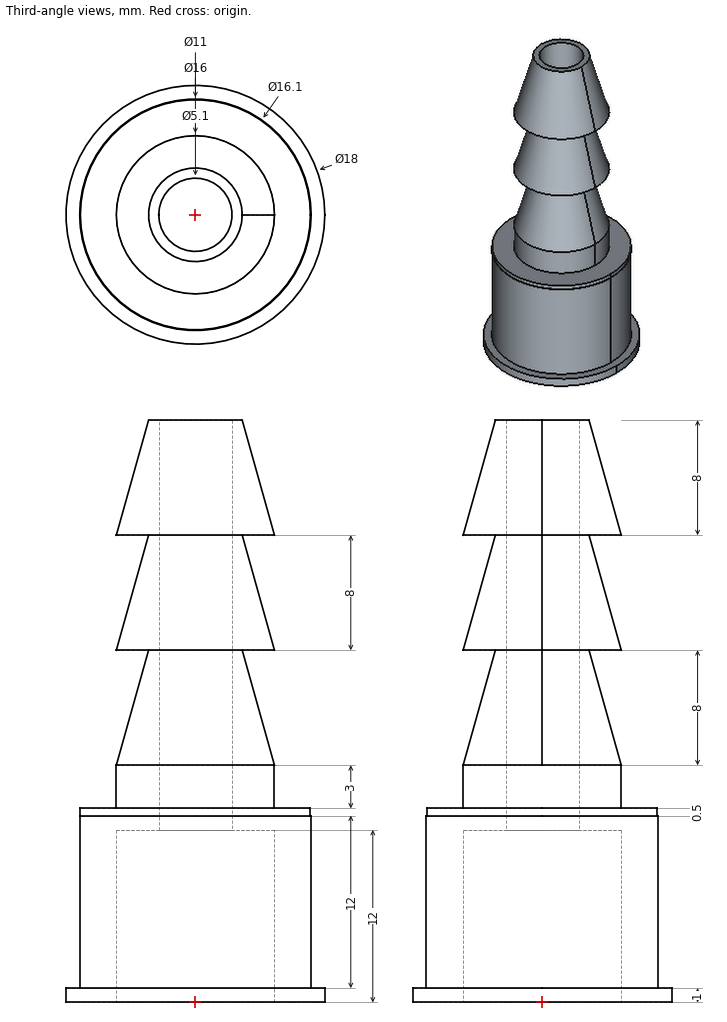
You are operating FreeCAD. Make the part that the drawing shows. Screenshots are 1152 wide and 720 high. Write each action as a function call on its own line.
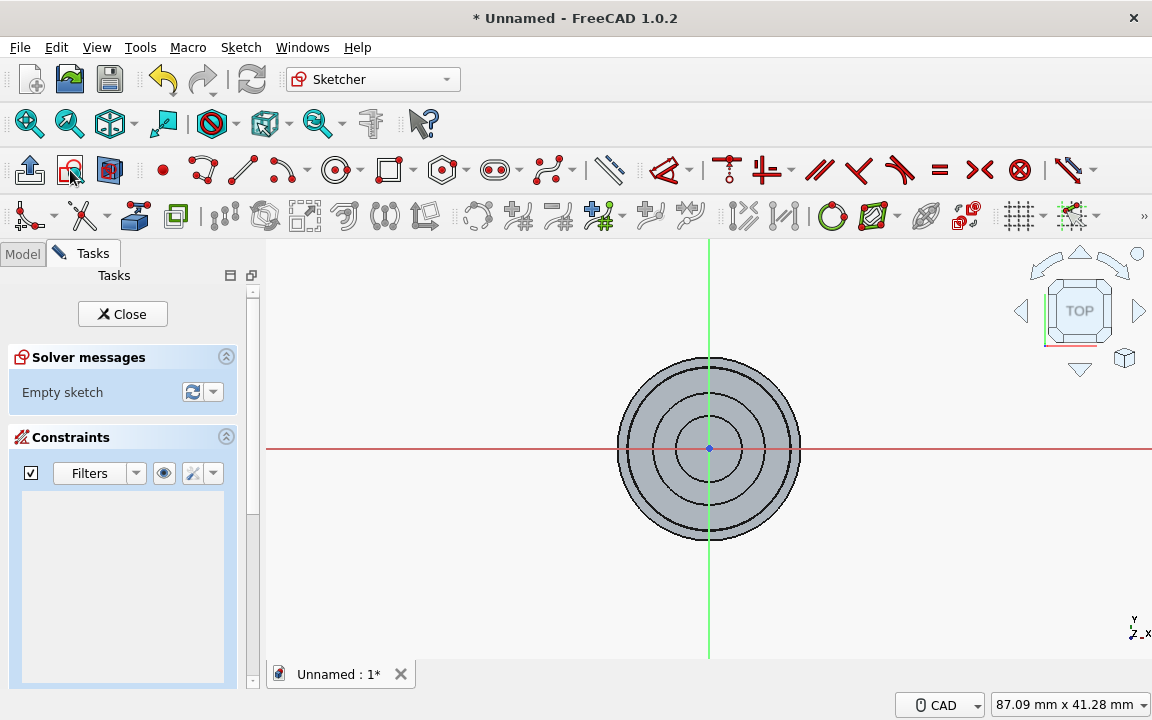
scroll(765, 449, up, 4)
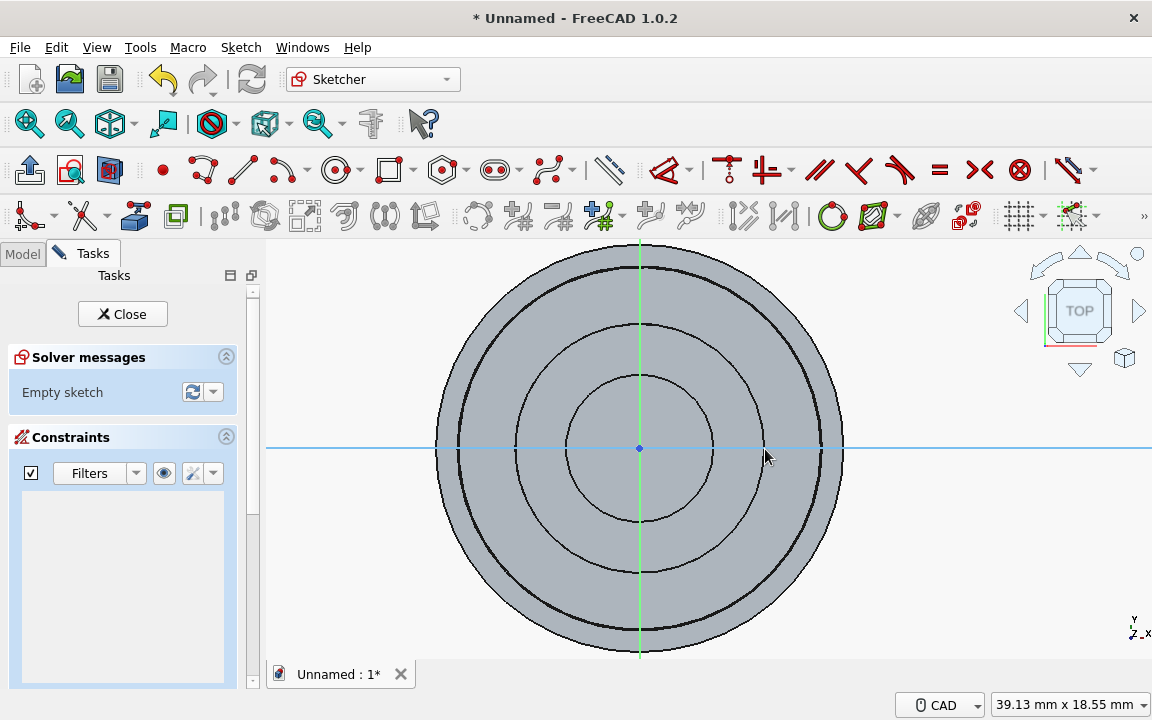
key(g)
key(c)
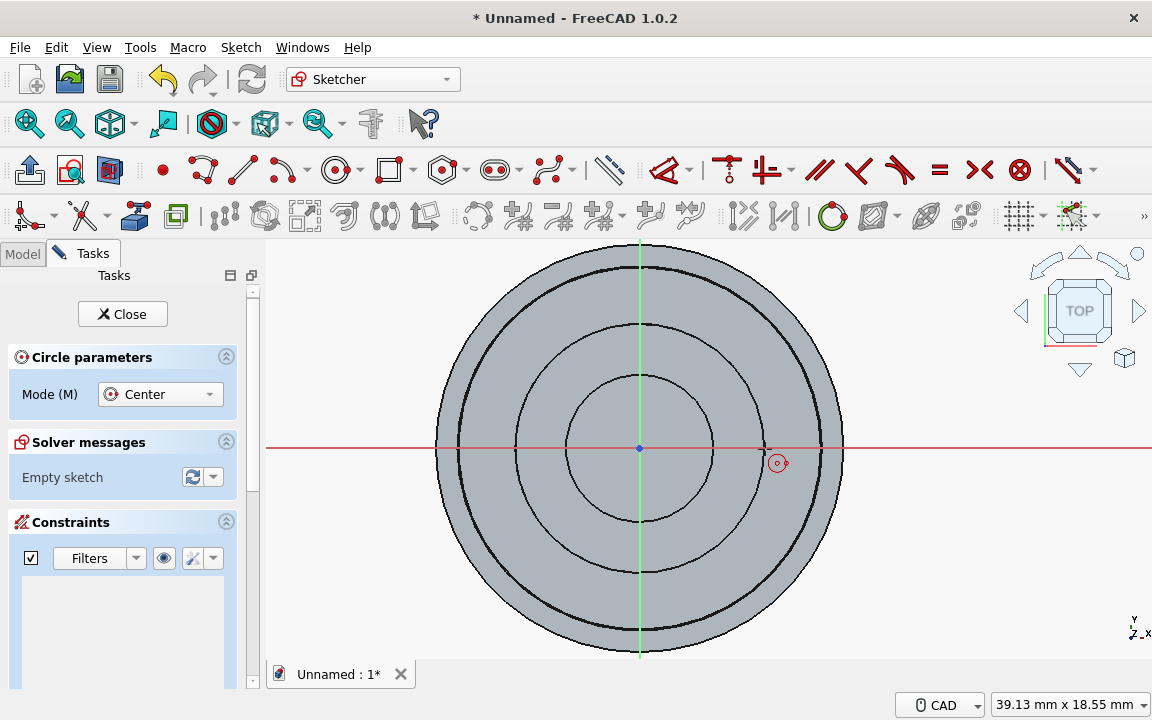
click(640, 448)
click(728, 360)
key(Escape)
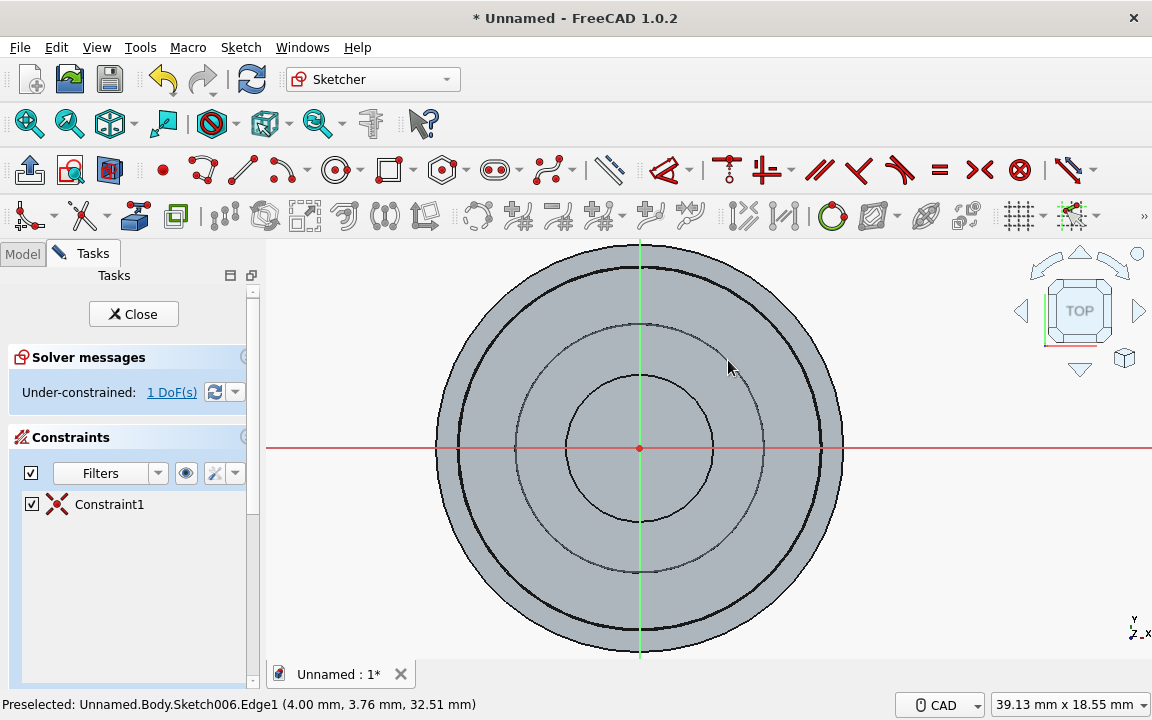
key(d)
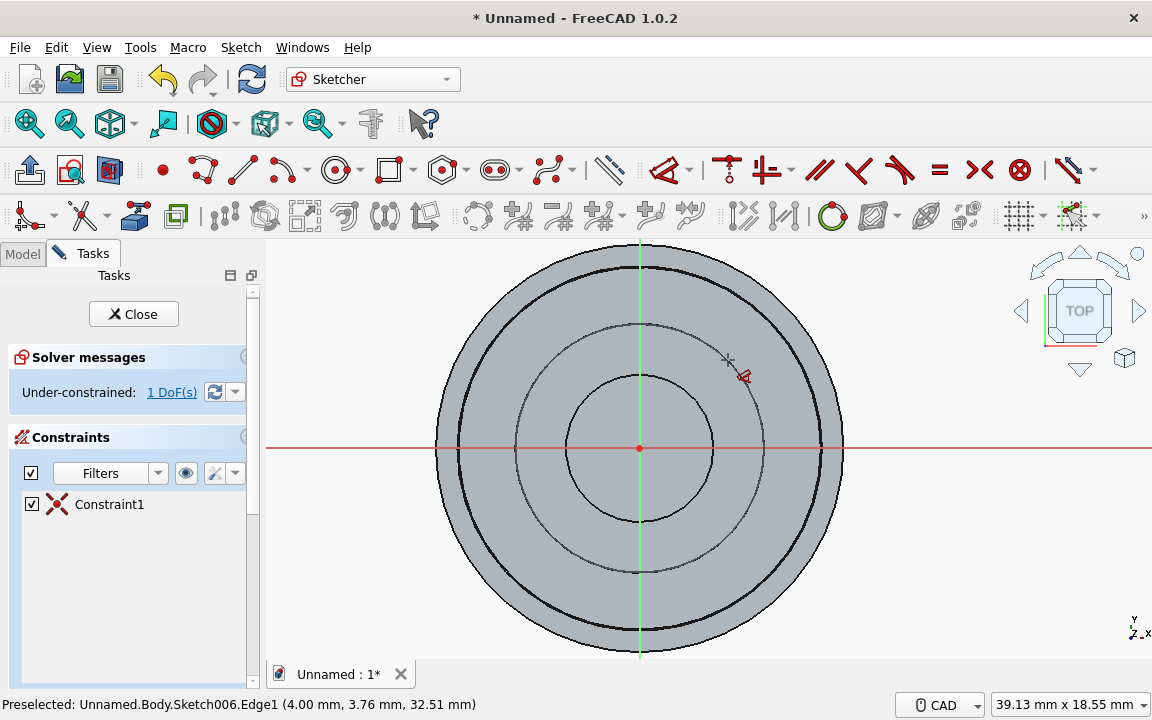
click(727, 360)
click(749, 337)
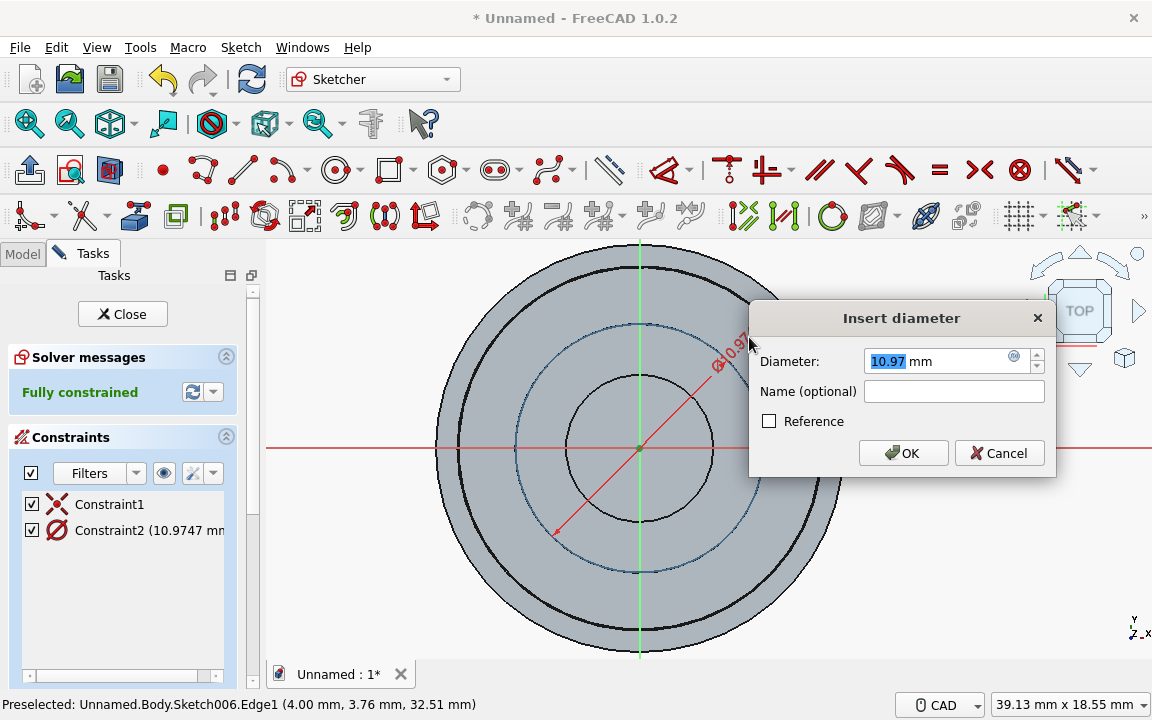
text(11)
key(Return)
key(Escape)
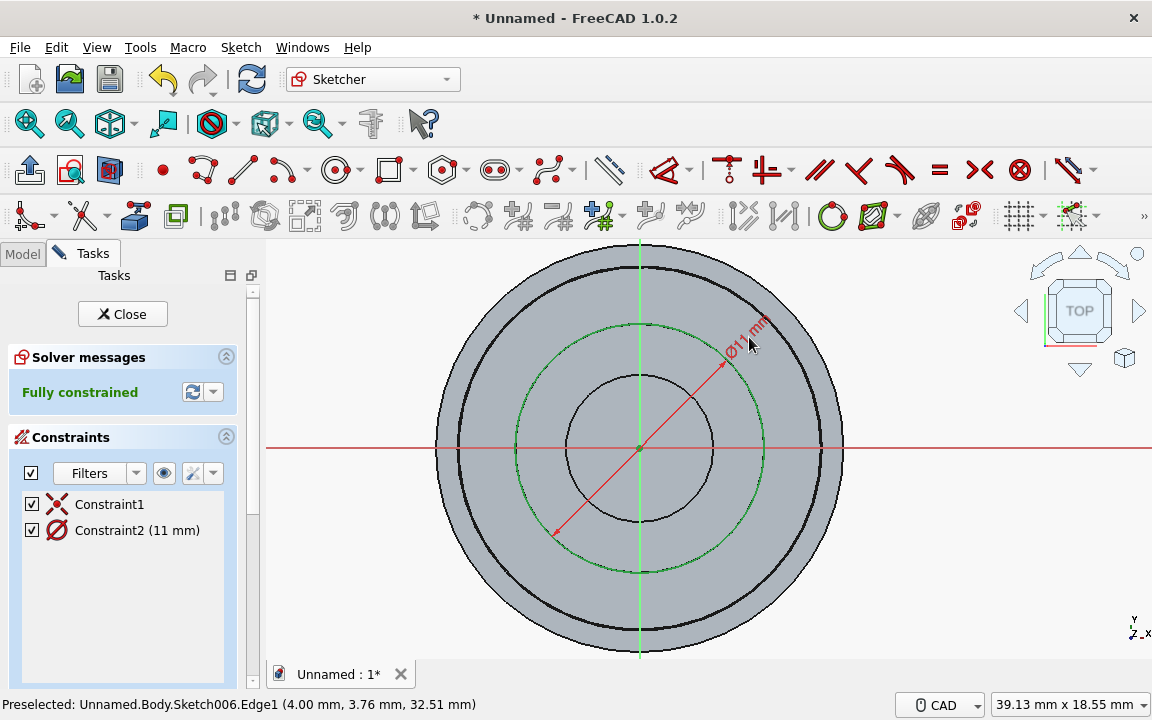
click(123, 314)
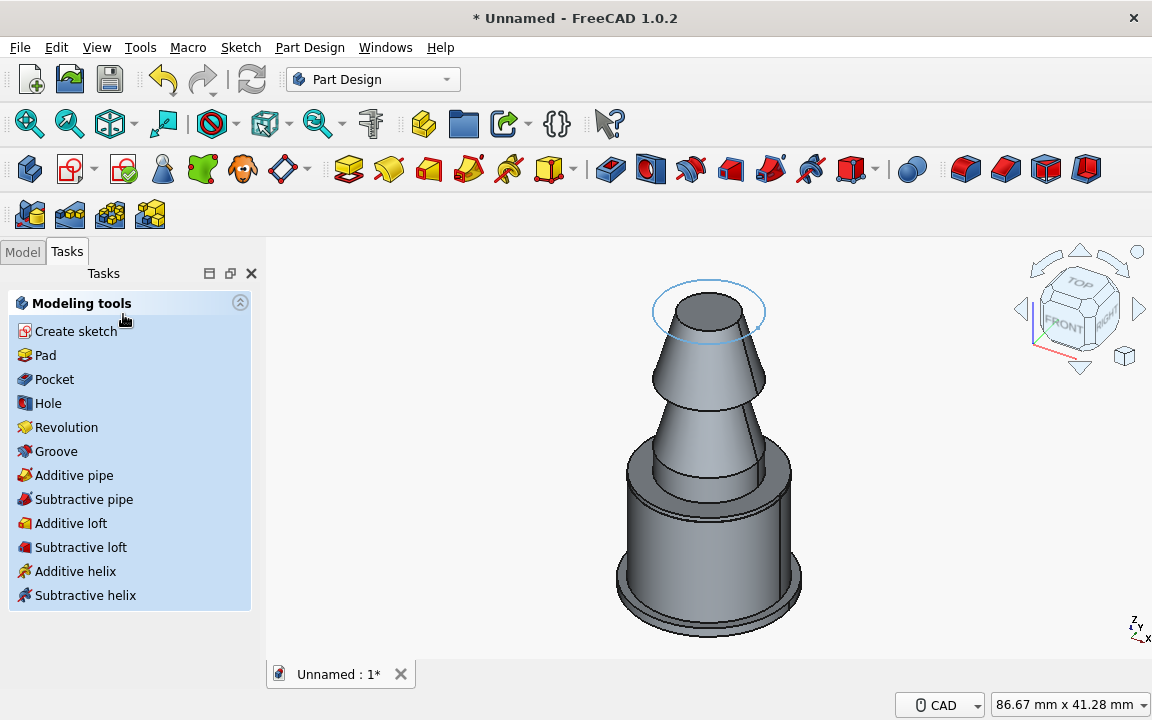
click(350, 170)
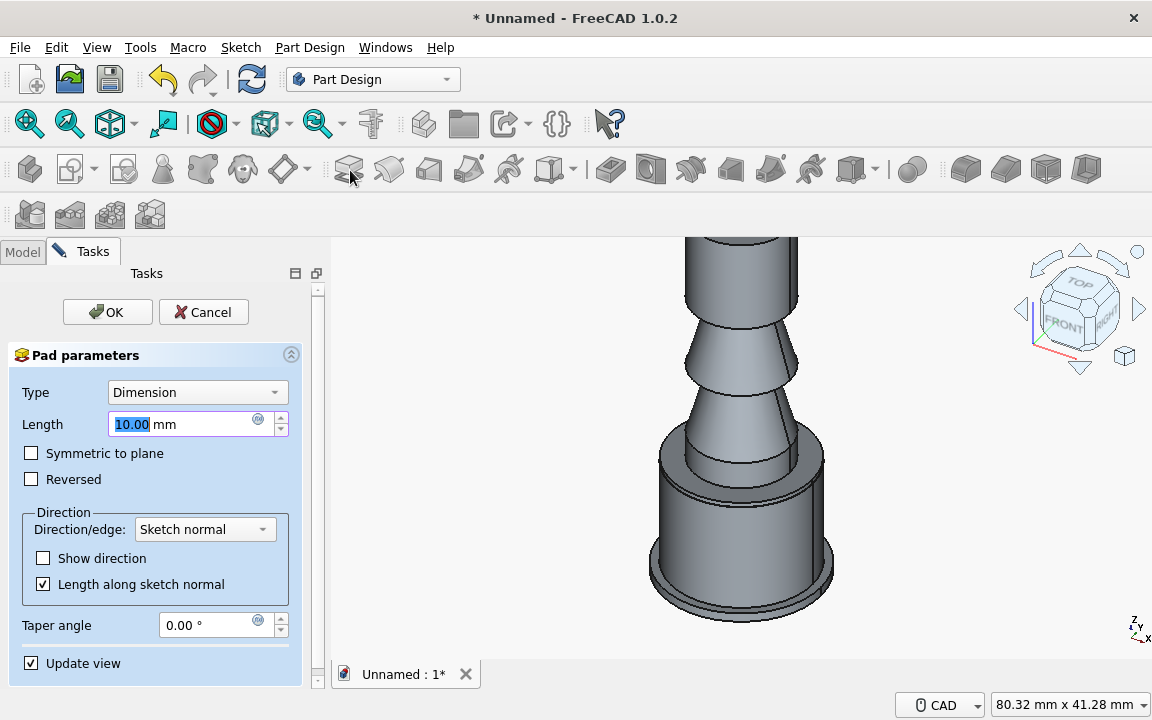
text(8)
key(Tab)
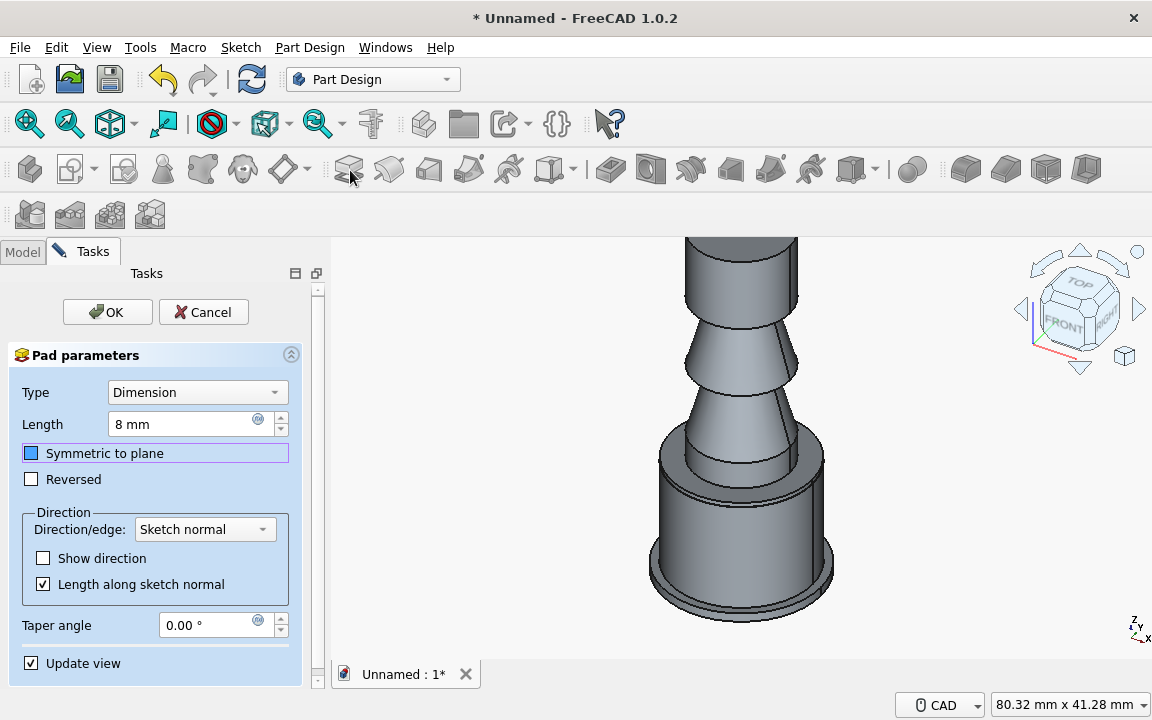
triple_click(216, 625)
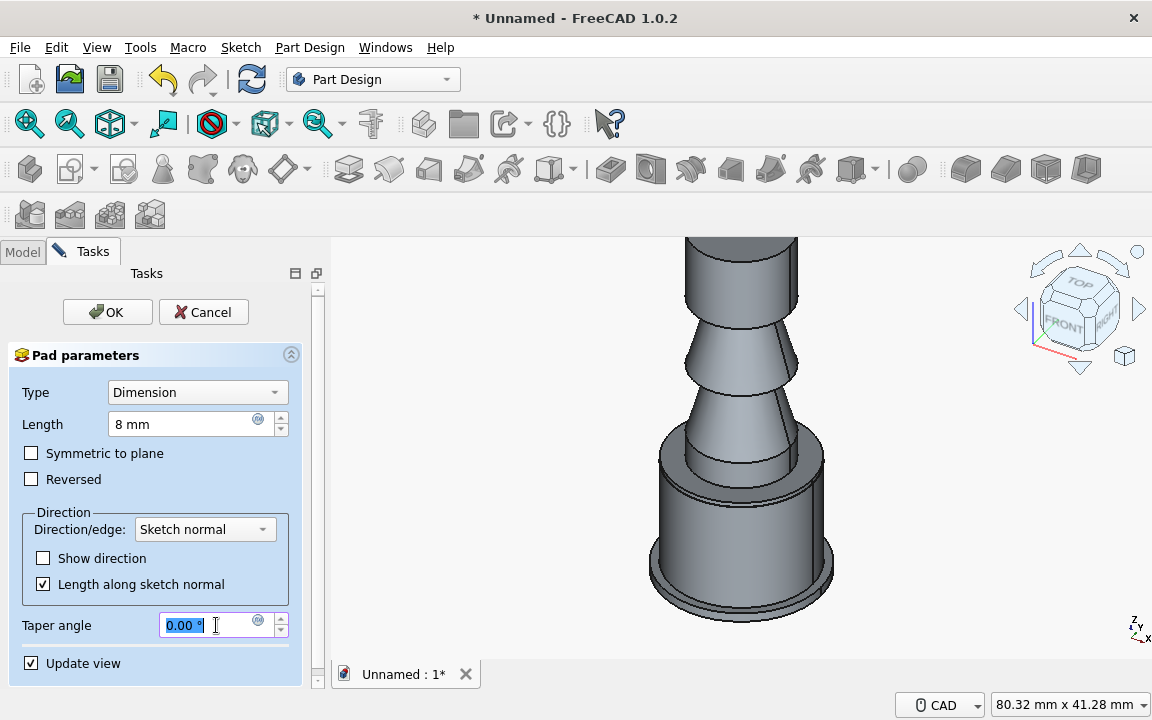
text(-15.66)
key(Tab)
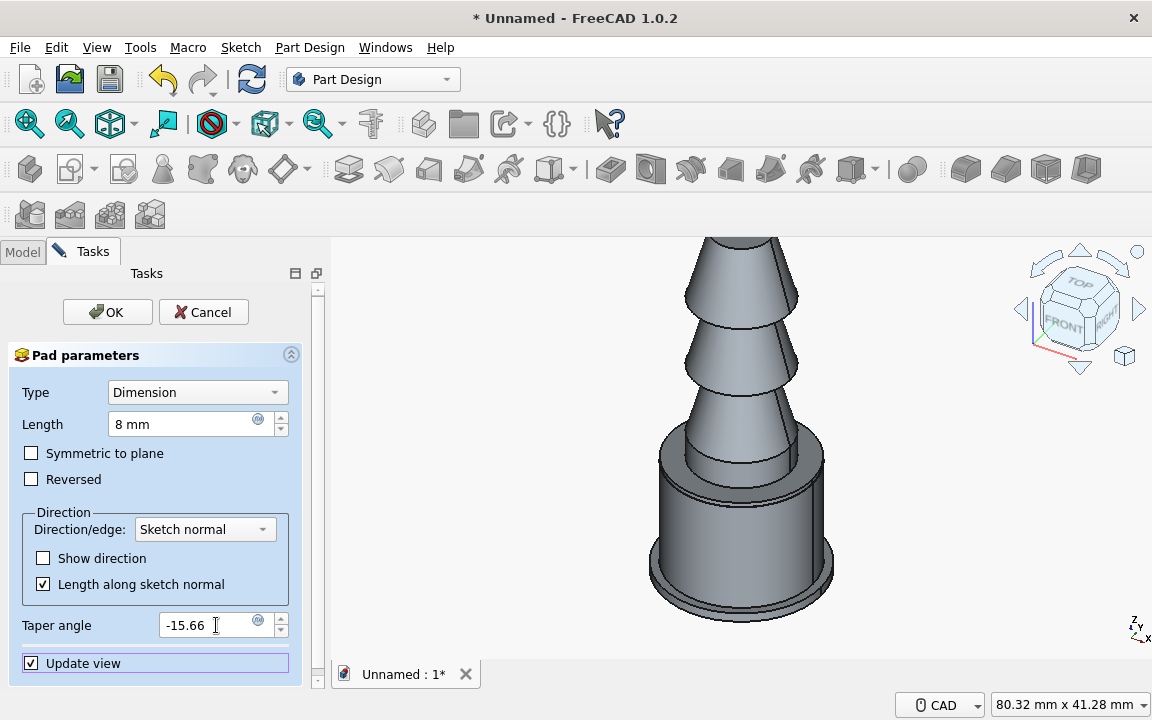
click(108, 312)